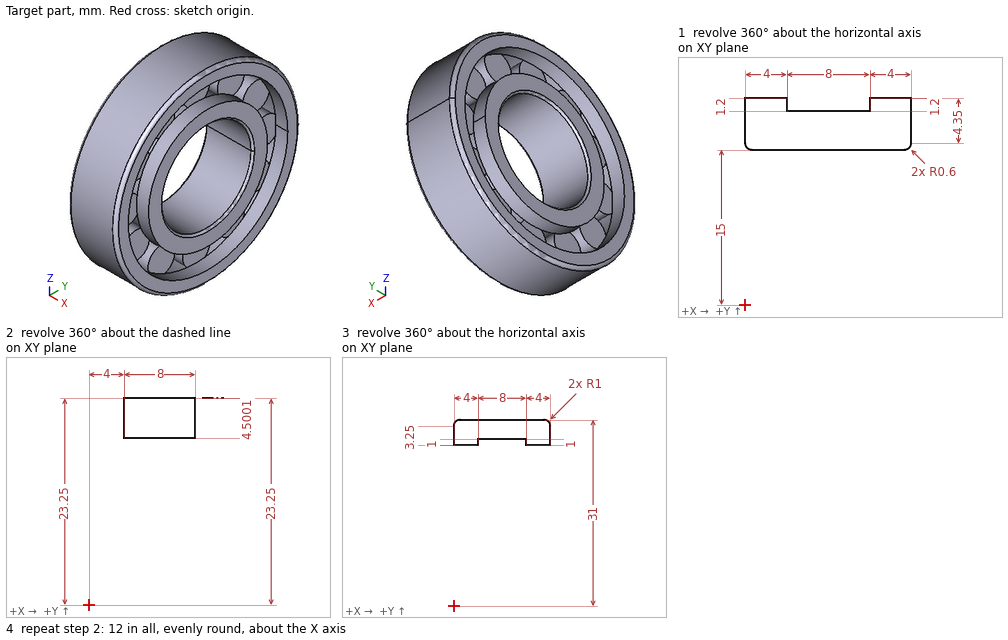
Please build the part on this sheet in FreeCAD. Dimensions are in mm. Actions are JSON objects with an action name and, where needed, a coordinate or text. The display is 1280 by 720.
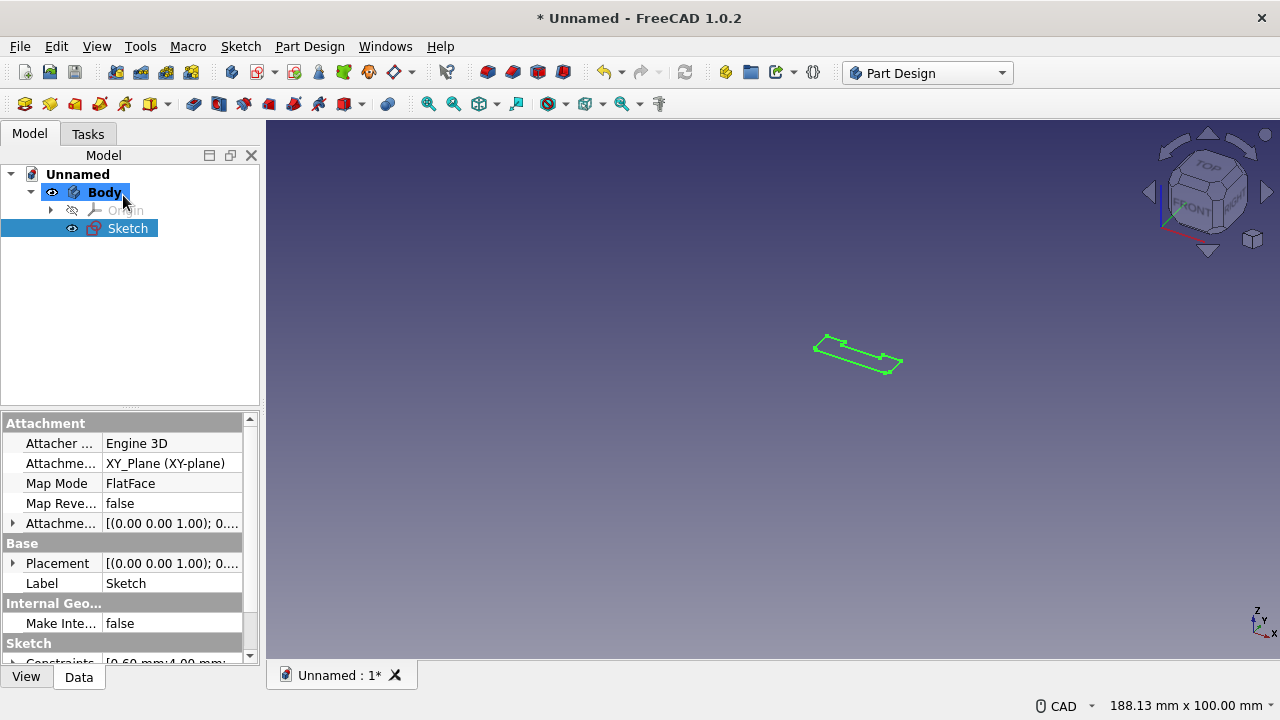
{"action": "left_click", "coordinate": [50, 104]}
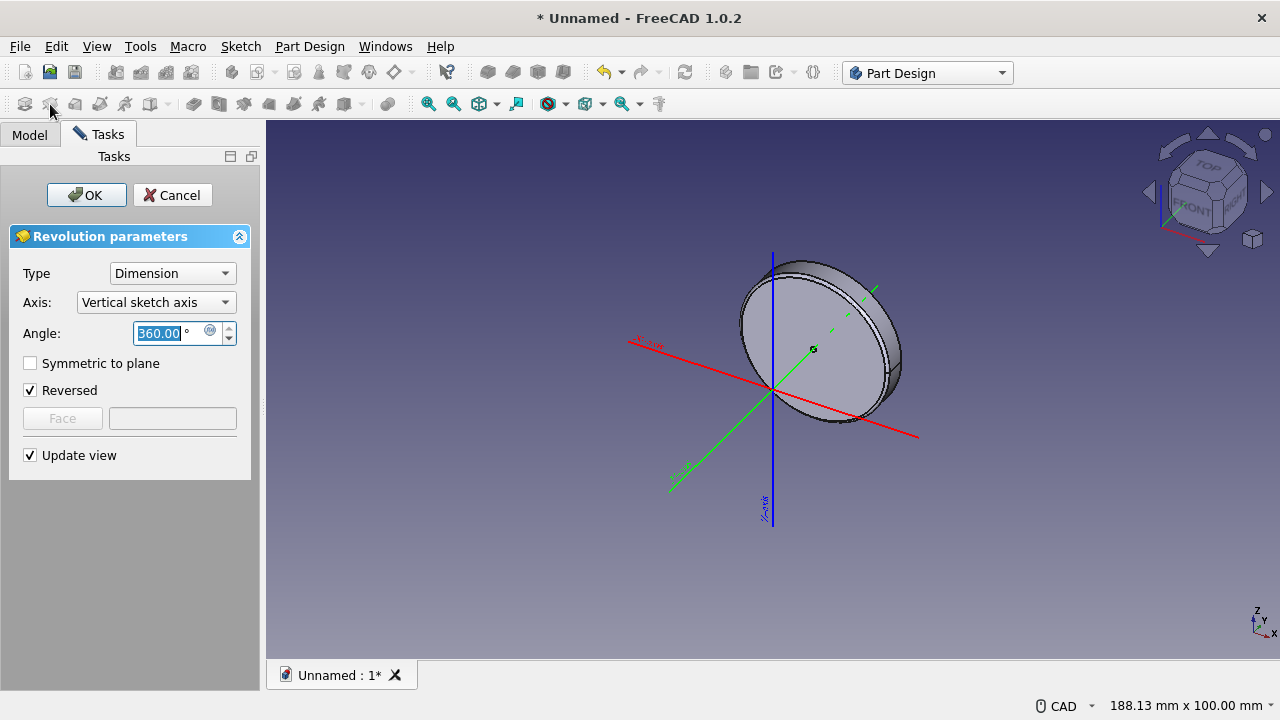
{"action": "left_click", "coordinate": [157, 302]}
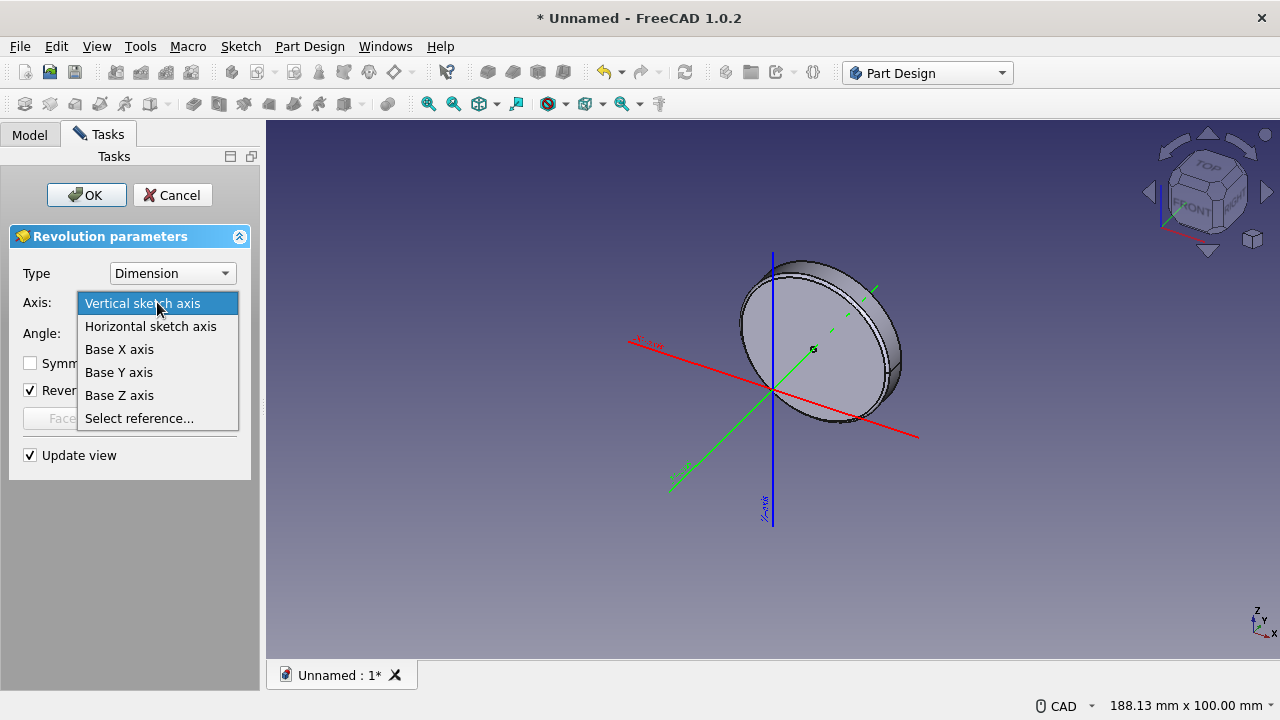
{"action": "left_click", "coordinate": [156, 326]}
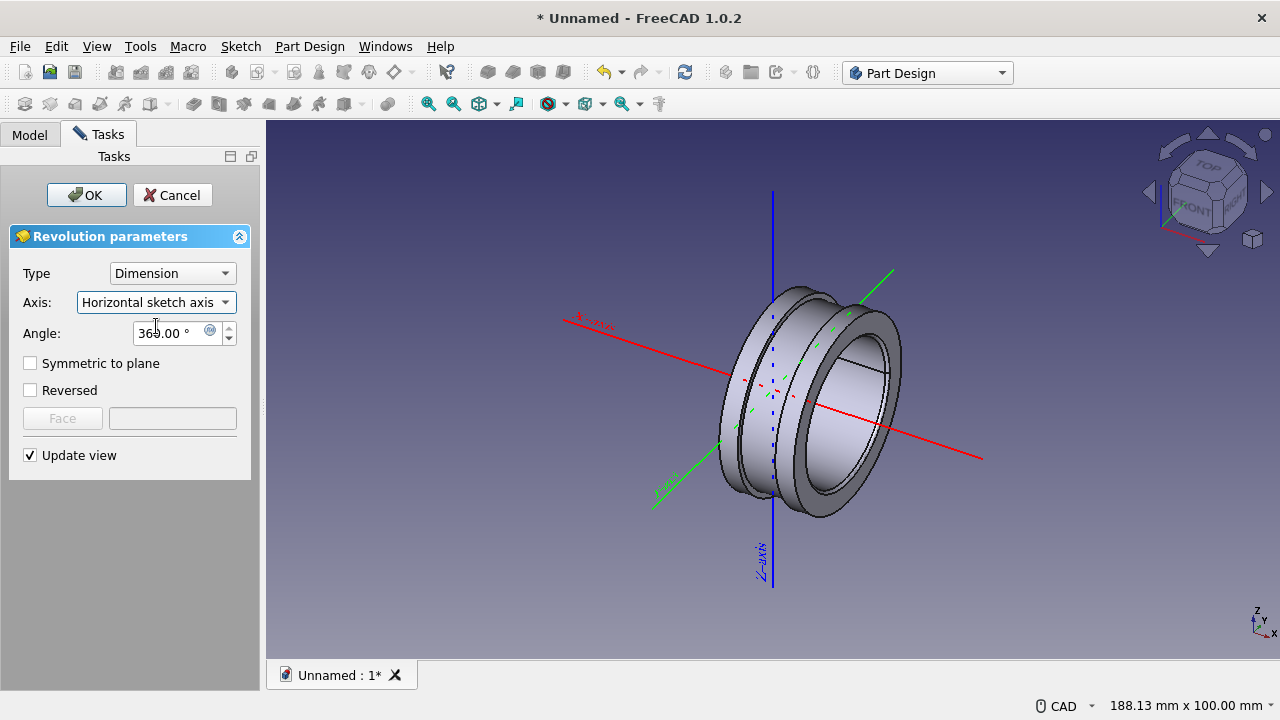
{"action": "left_click", "coordinate": [87, 195]}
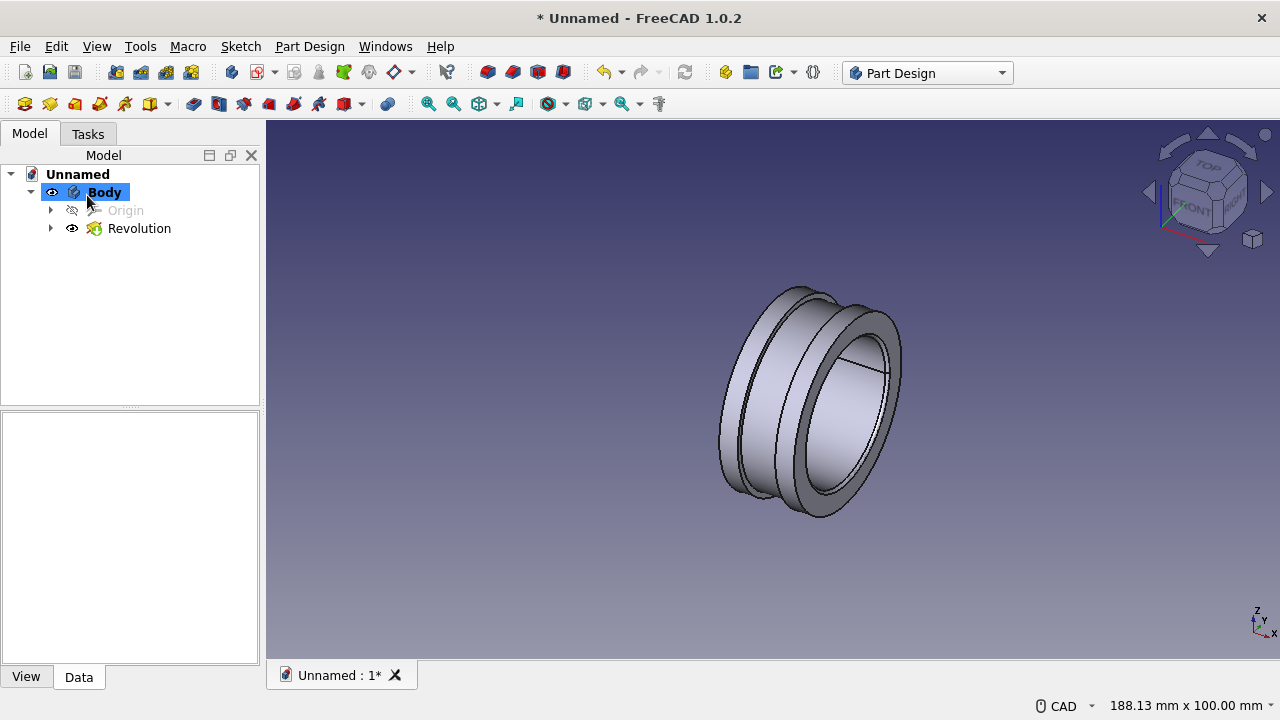
{"action": "left_click", "coordinate": [256, 72]}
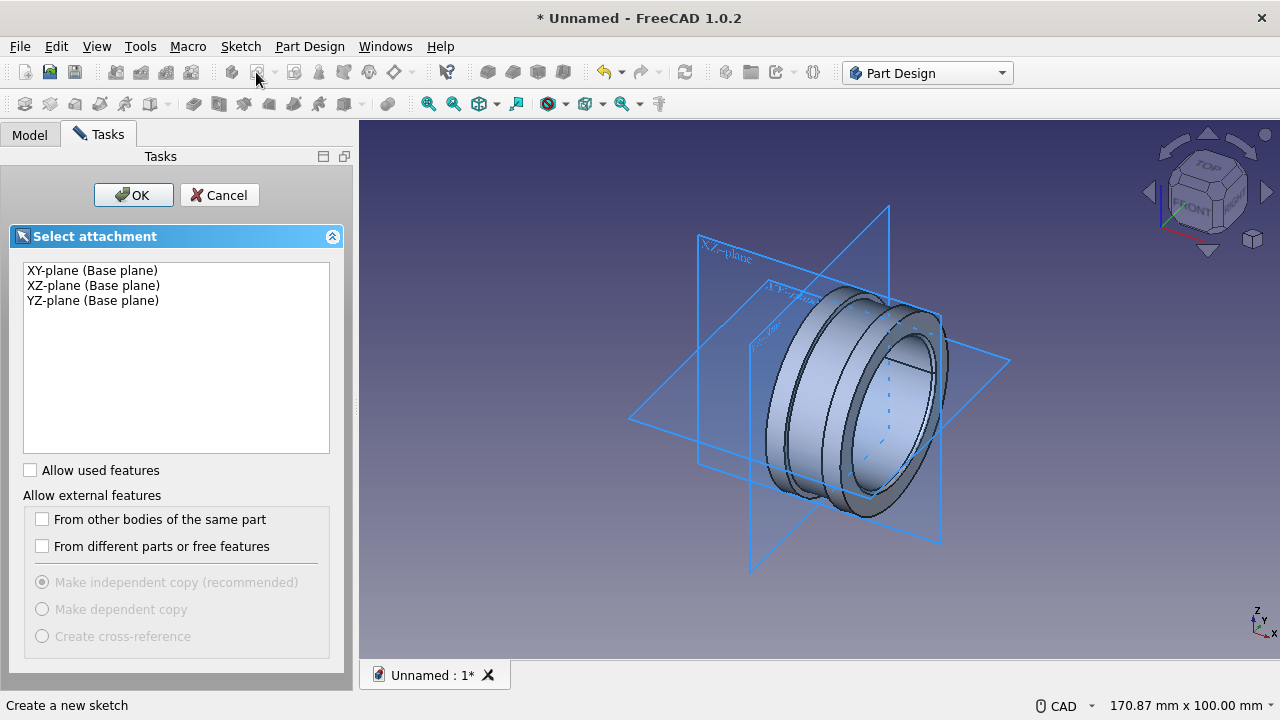
{"action": "left_click", "coordinate": [84, 270]}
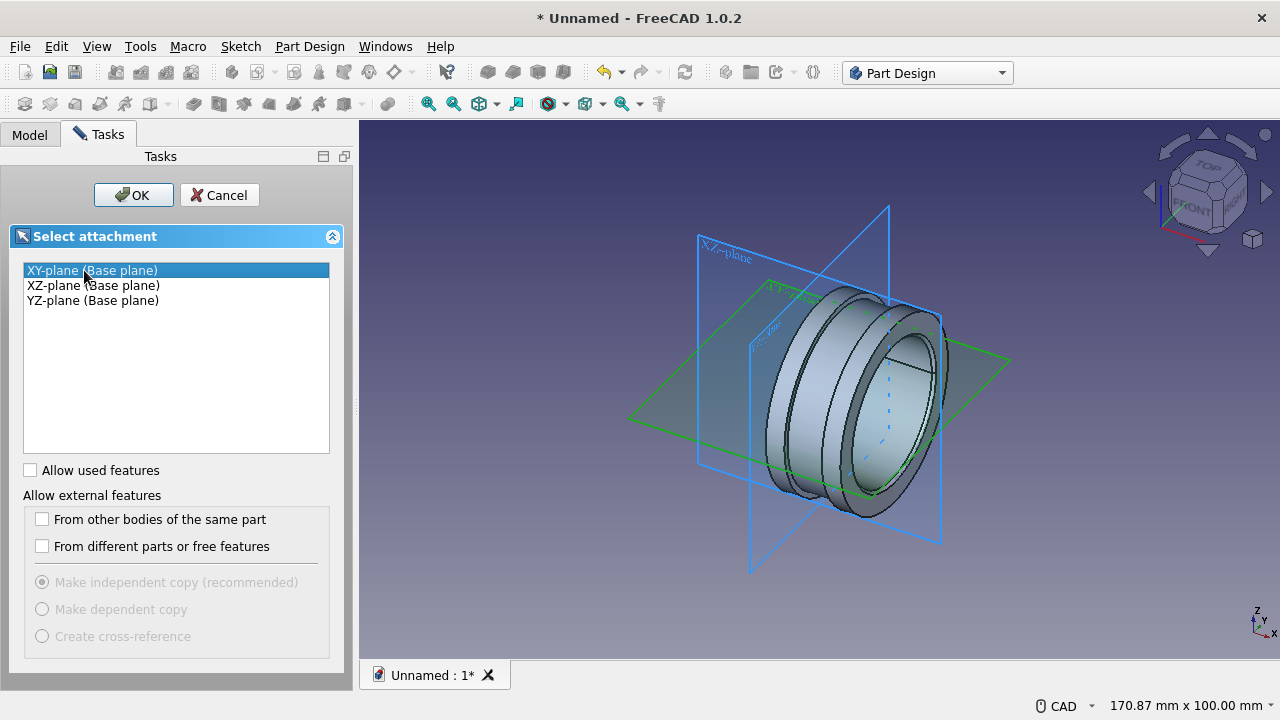
{"action": "left_click", "coordinate": [134, 195]}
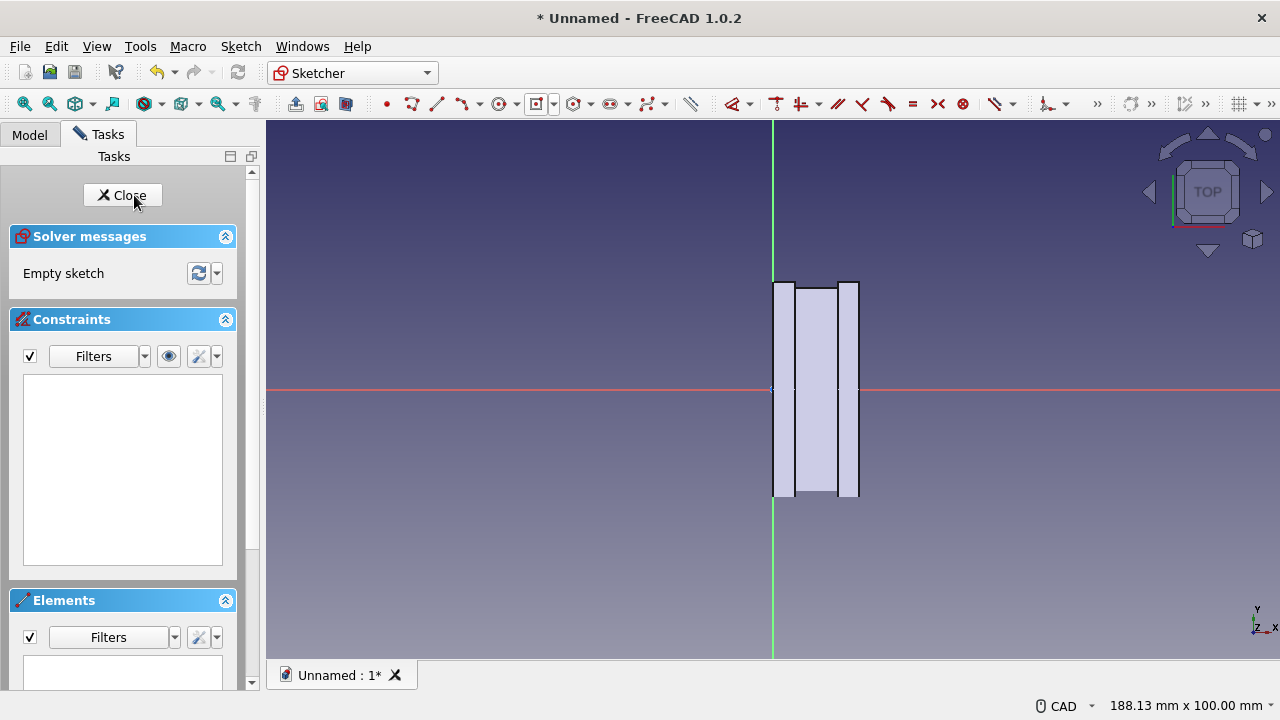
{"action": "left_click", "coordinate": [346, 104]}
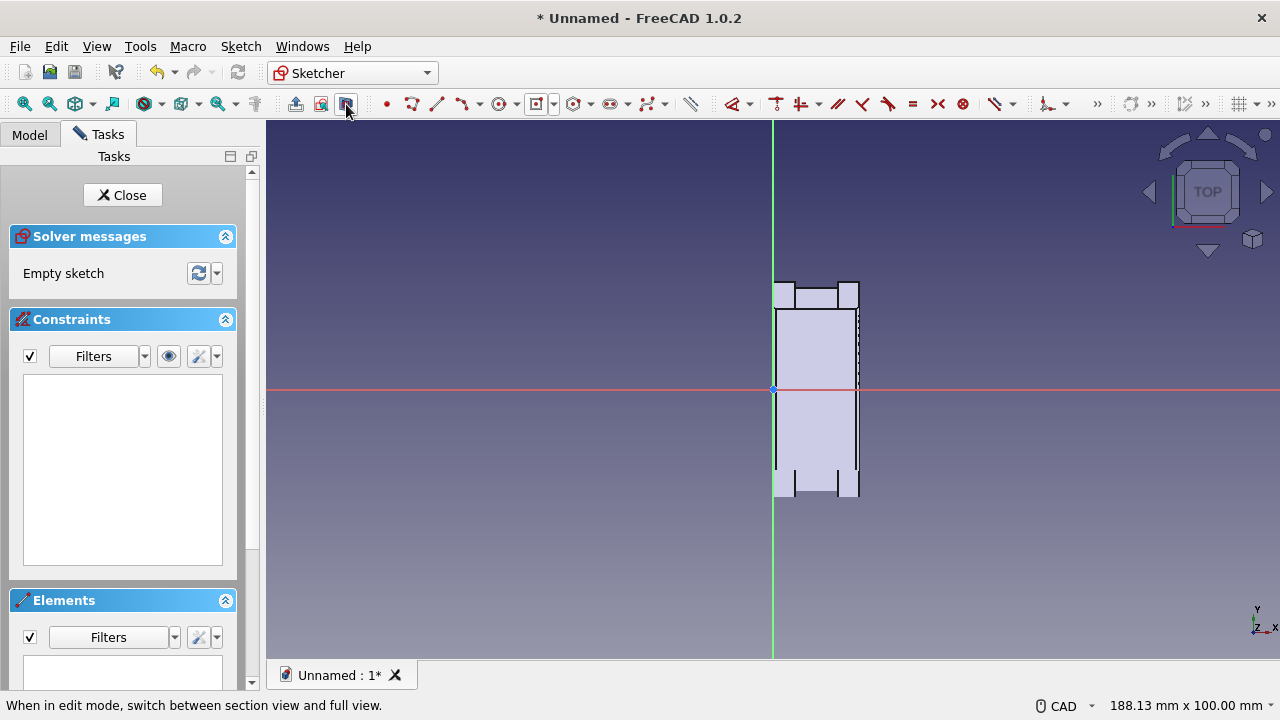
{"action": "scroll", "coordinate": [878, 290], "scroll_direction": "up", "scroll_amount": 5}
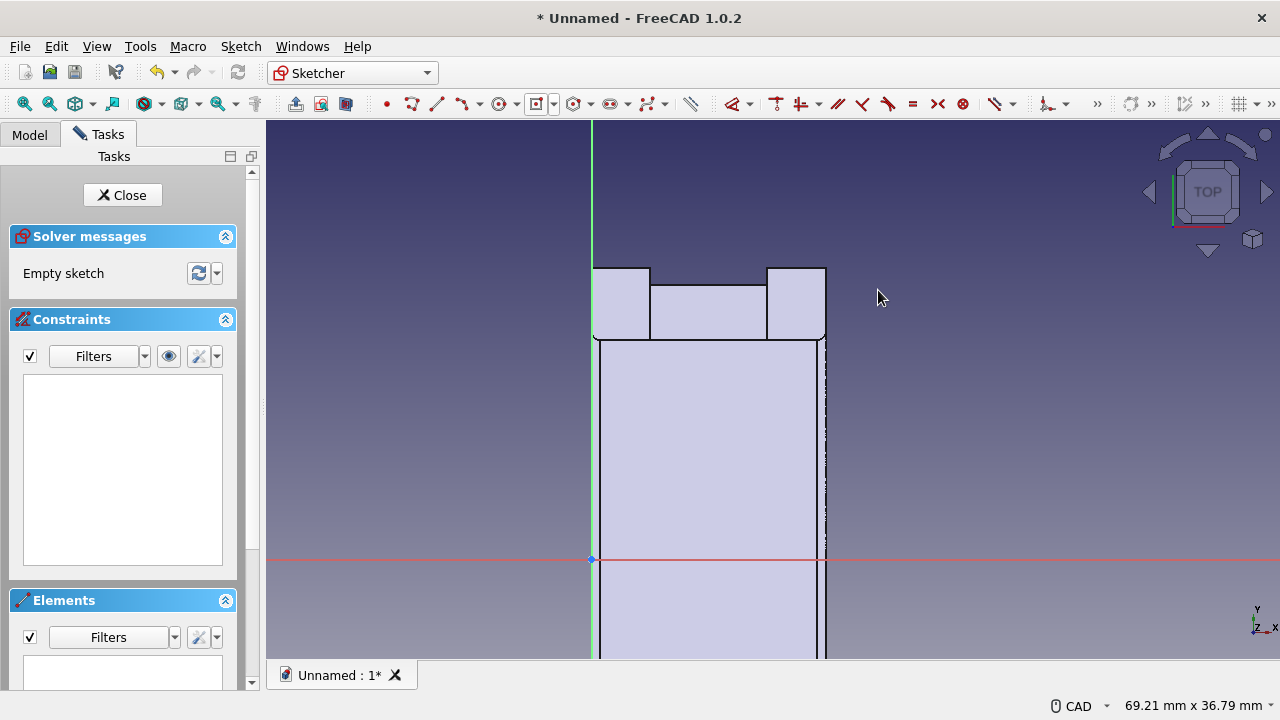
{"action": "left_click", "coordinate": [554, 104]}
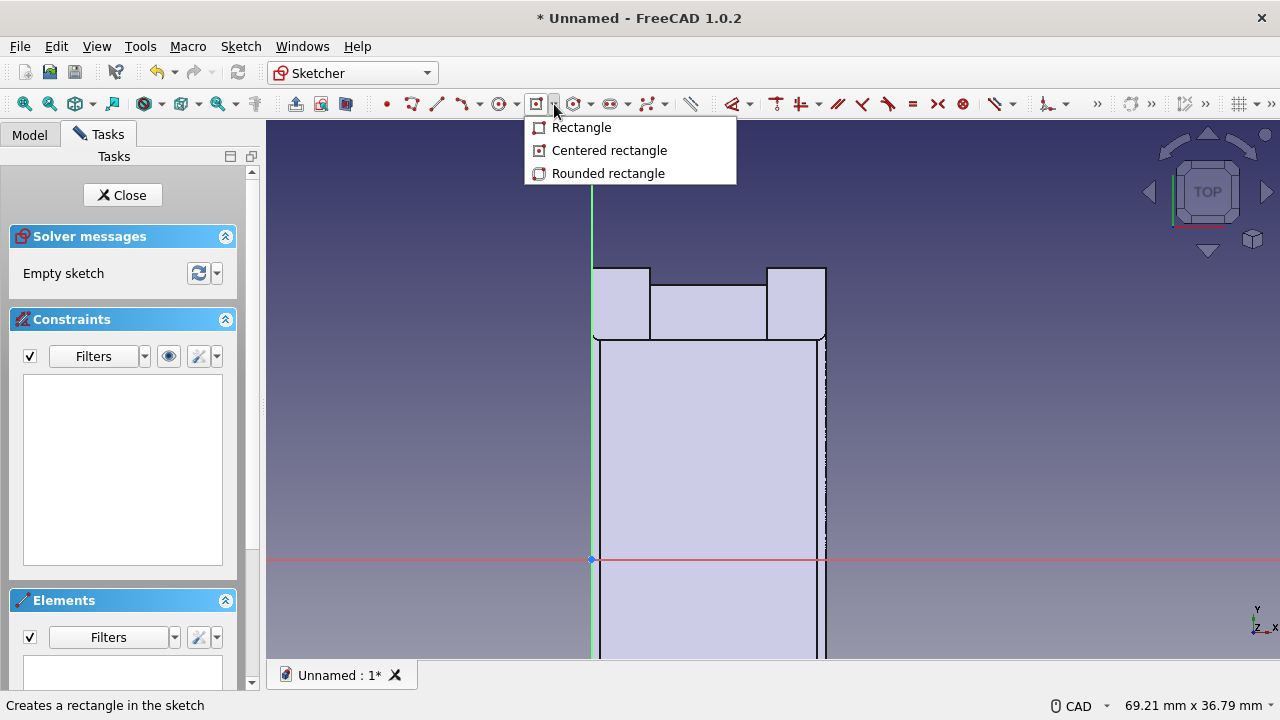
{"action": "left_click", "coordinate": [630, 128]}